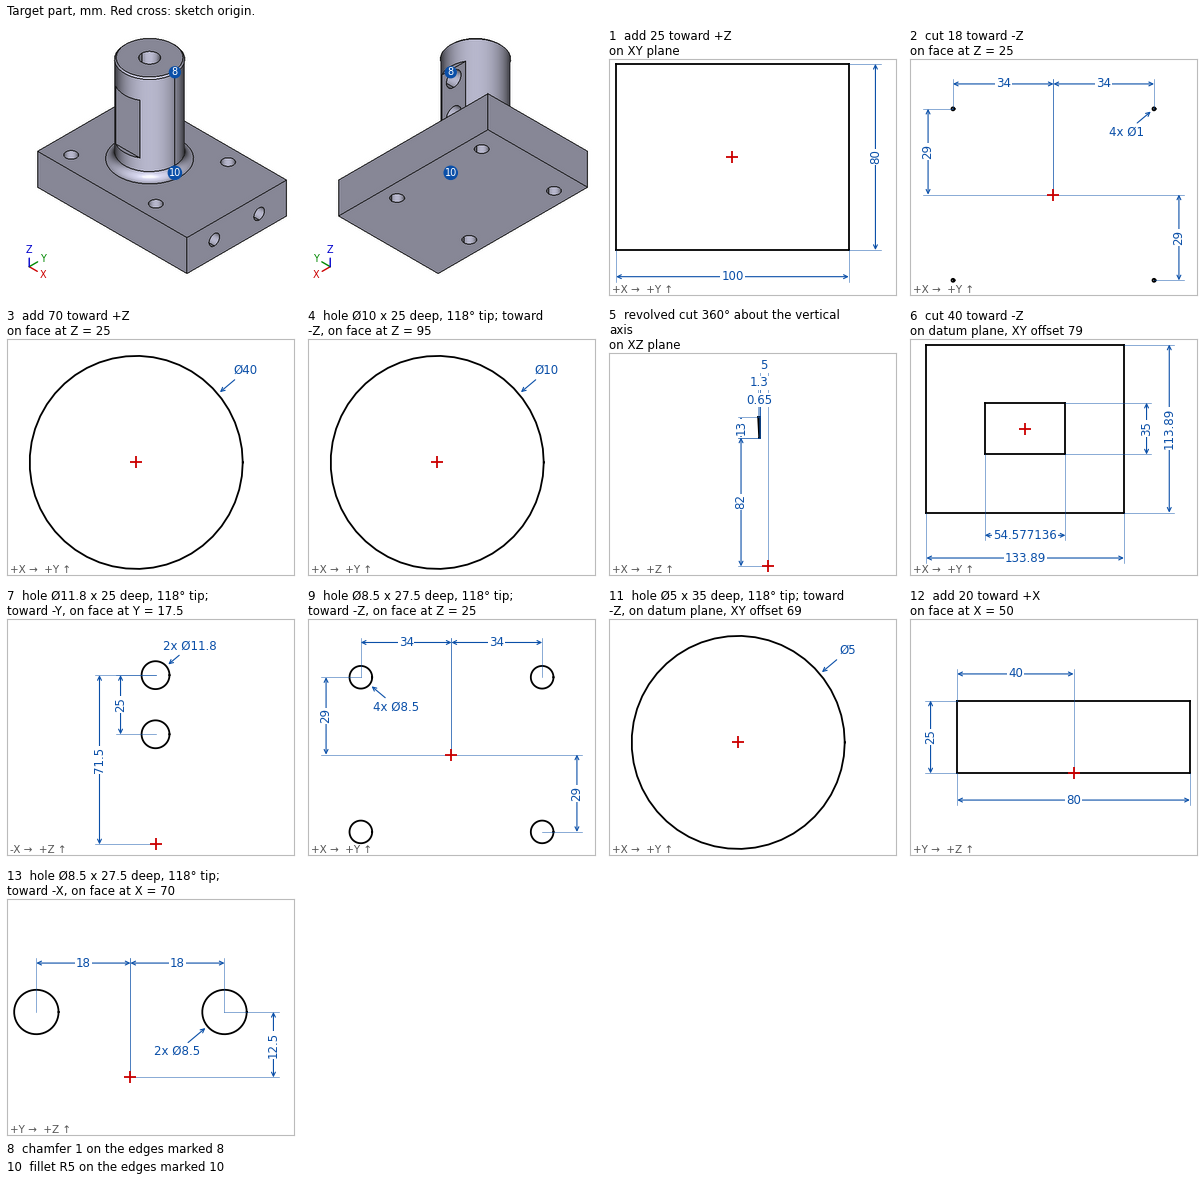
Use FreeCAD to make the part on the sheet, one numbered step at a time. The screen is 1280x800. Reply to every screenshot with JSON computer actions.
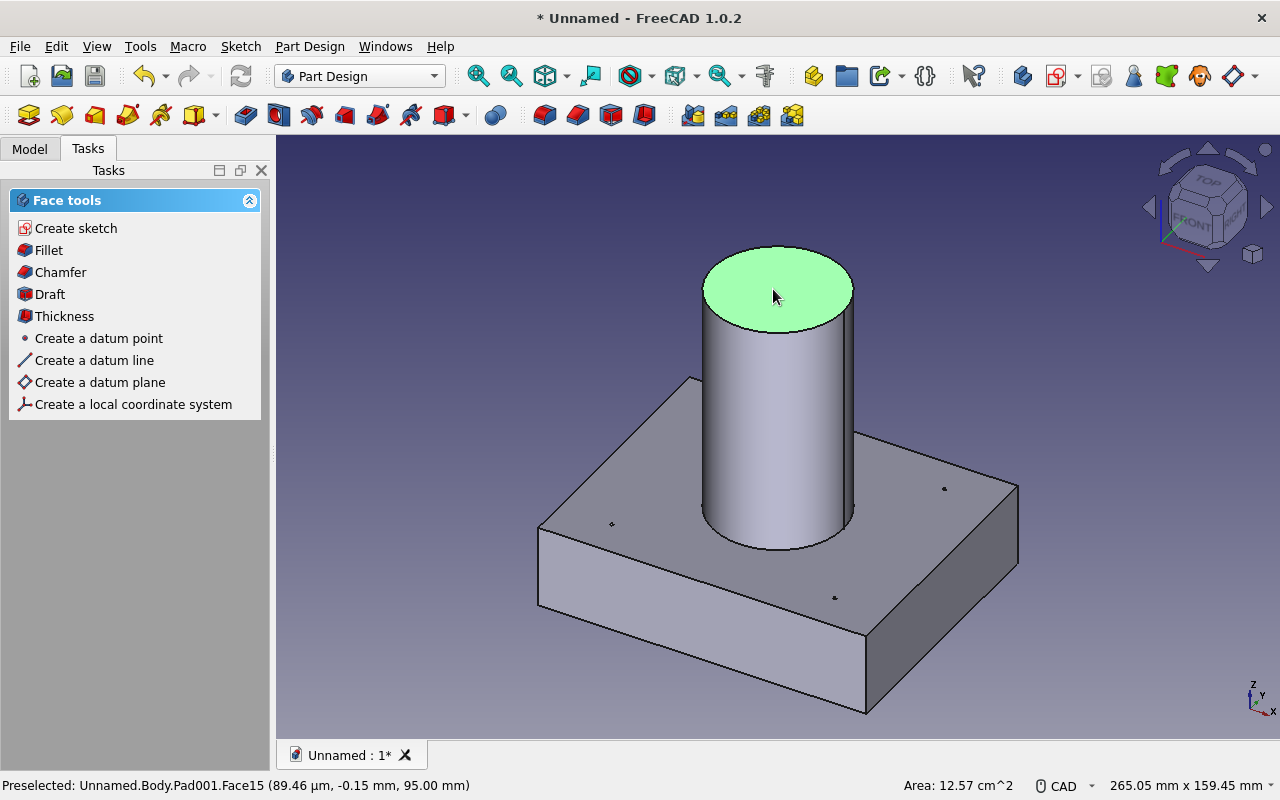
{"action": "left_click", "coordinate": [1056, 76]}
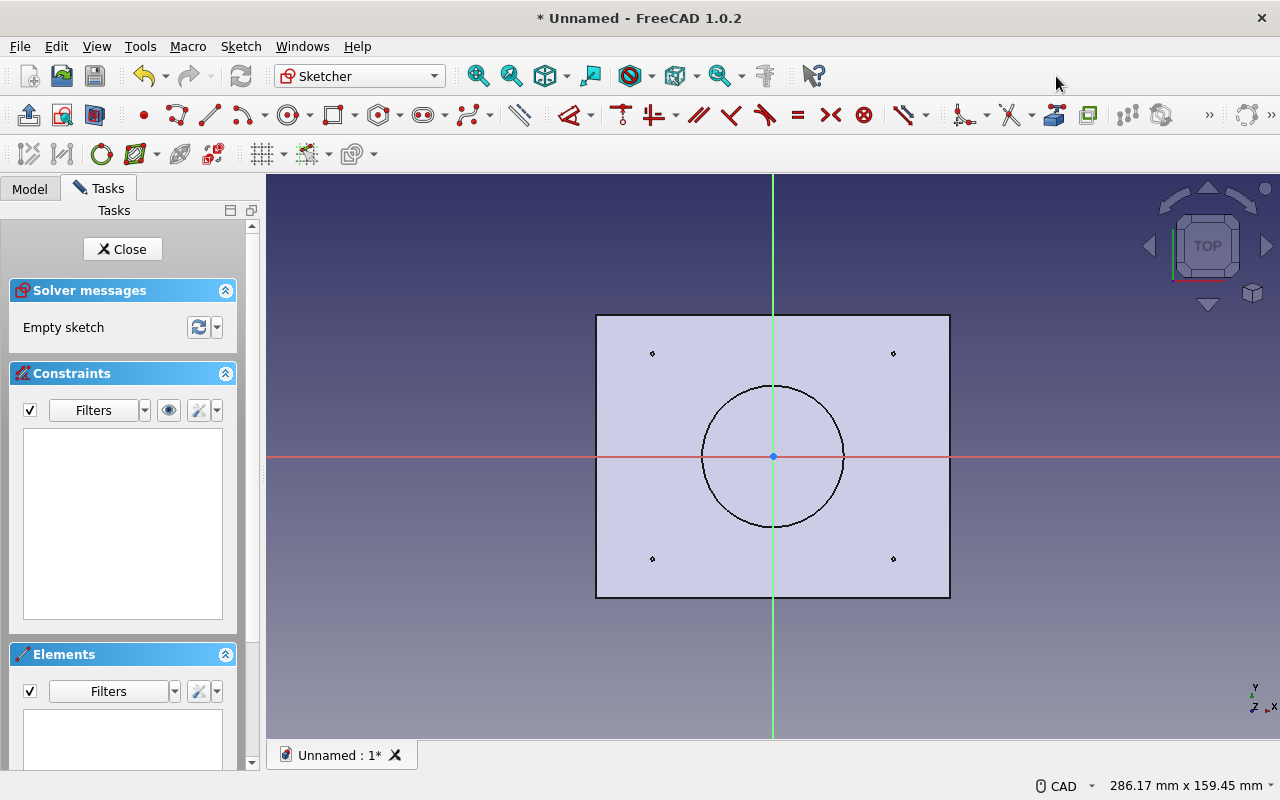
{"action": "scroll", "coordinate": [780, 456], "scroll_direction": "up", "scroll_amount": 12}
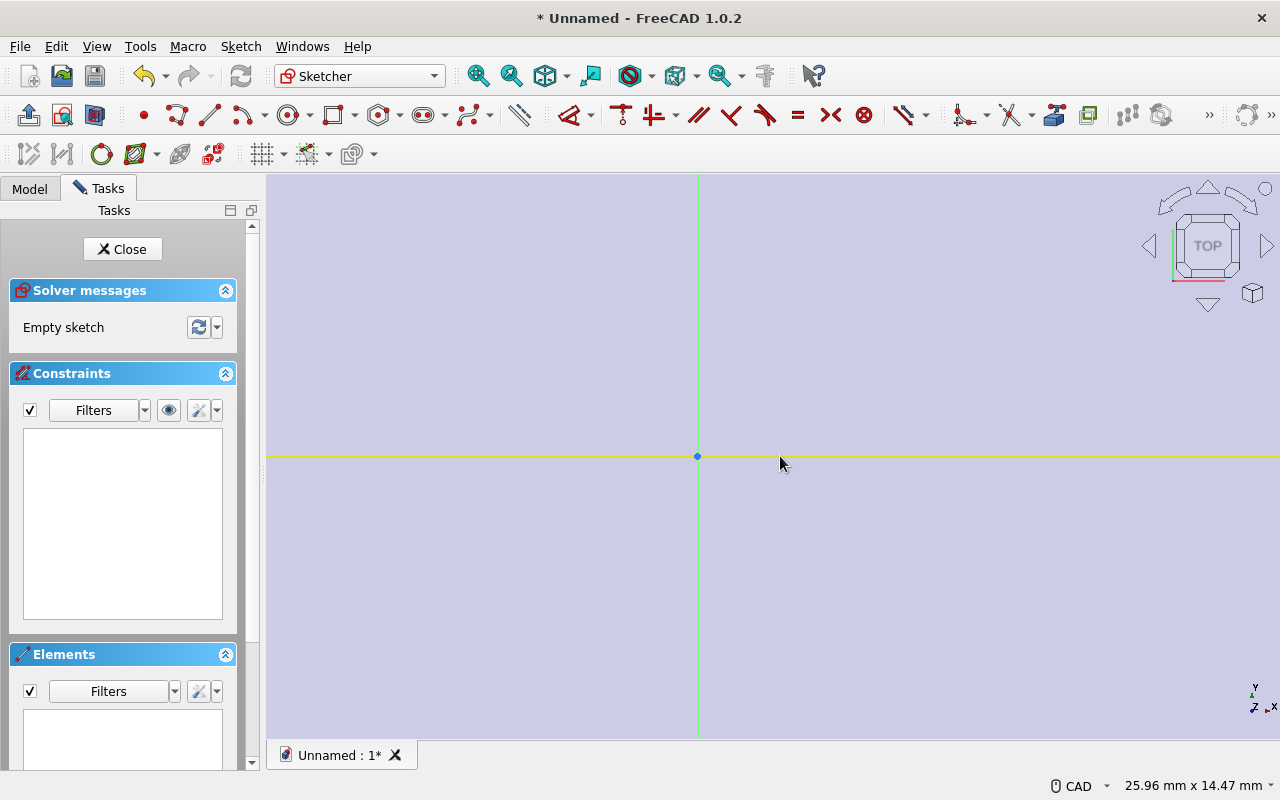
{"action": "key", "text": "g c"}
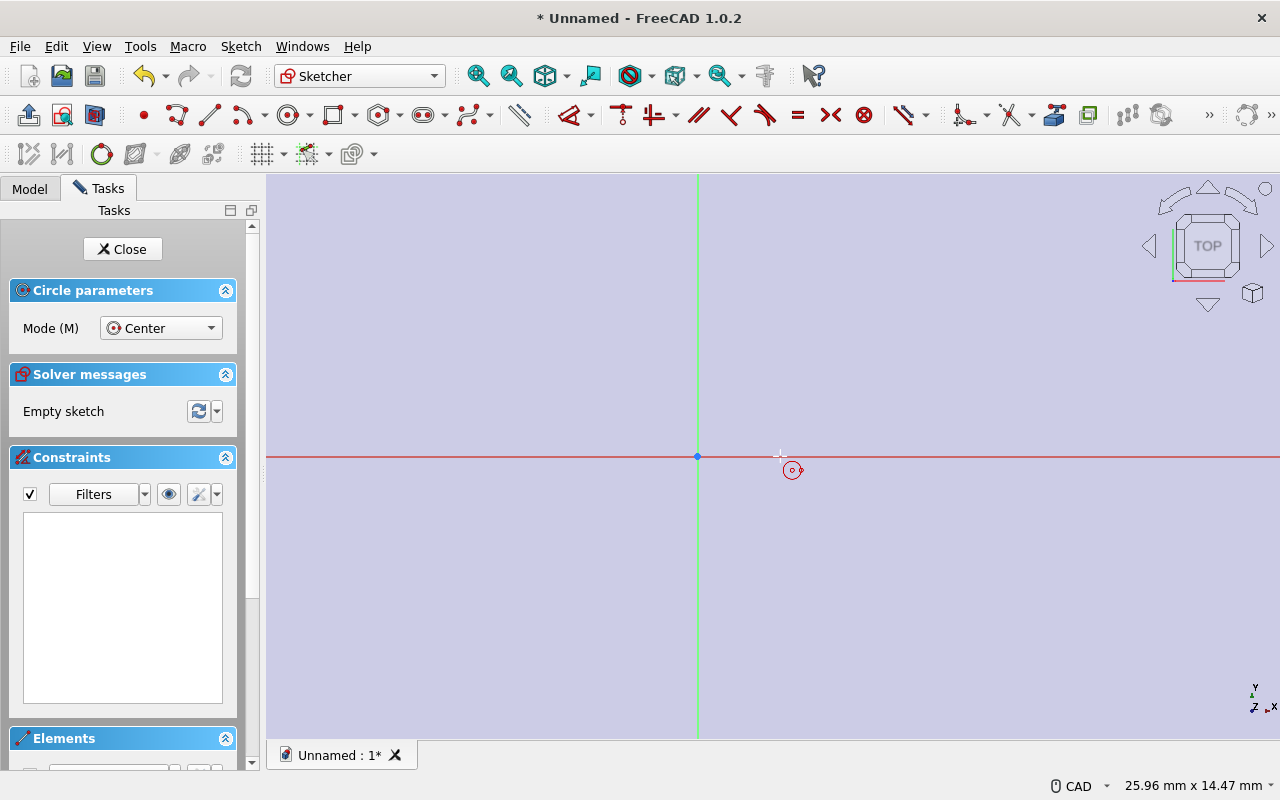
{"action": "left_click", "coordinate": [698, 456]}
{"action": "mouse_move", "coordinate": [836, 318]}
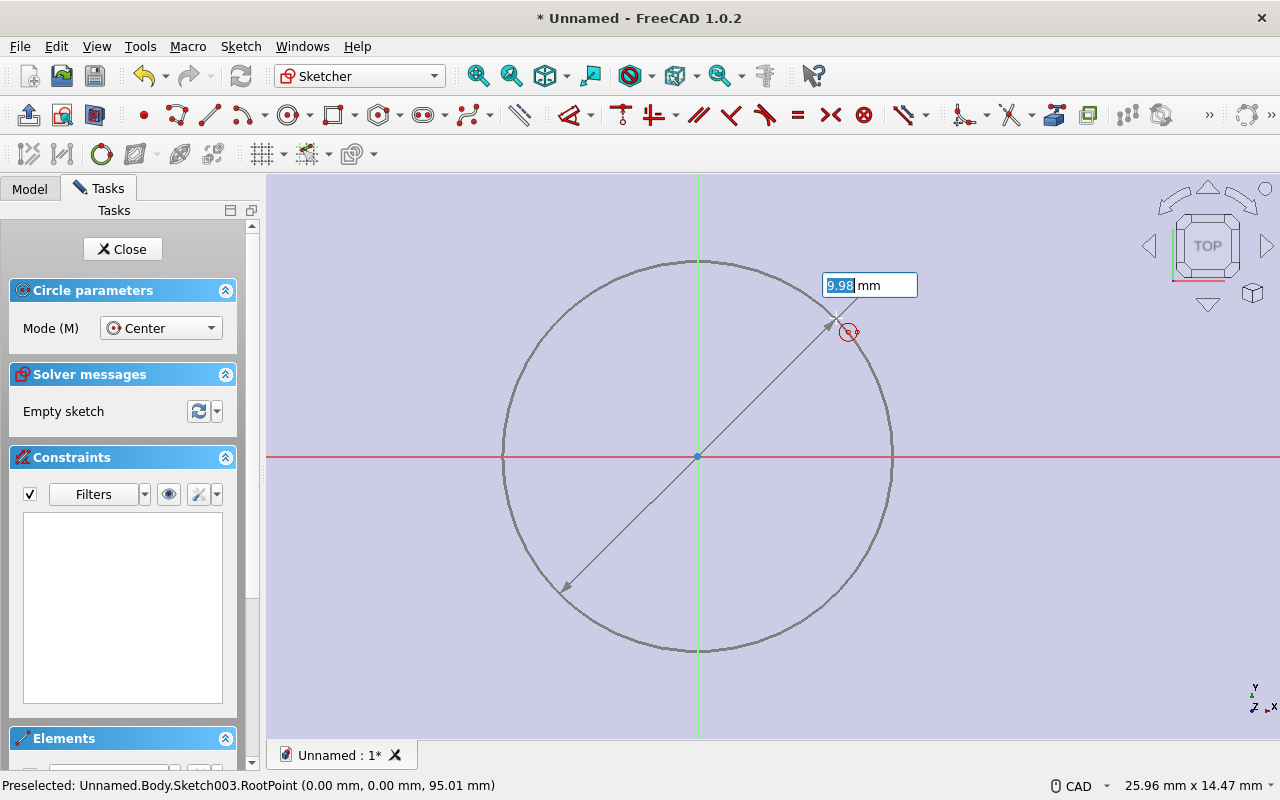
{"action": "type", "text": "10"}
{"action": "key", "text": "Return"}
{"action": "key", "text": "Escape"}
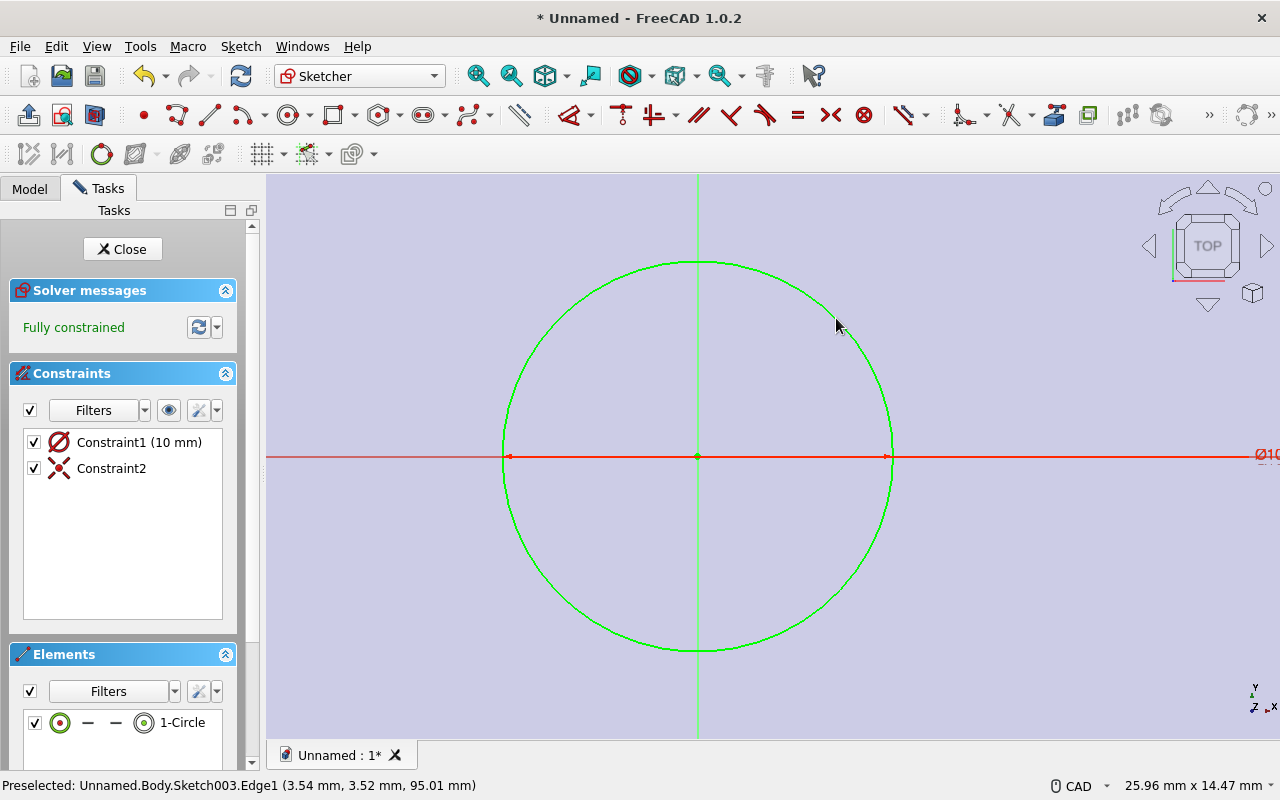
{"action": "left_click", "coordinate": [123, 249]}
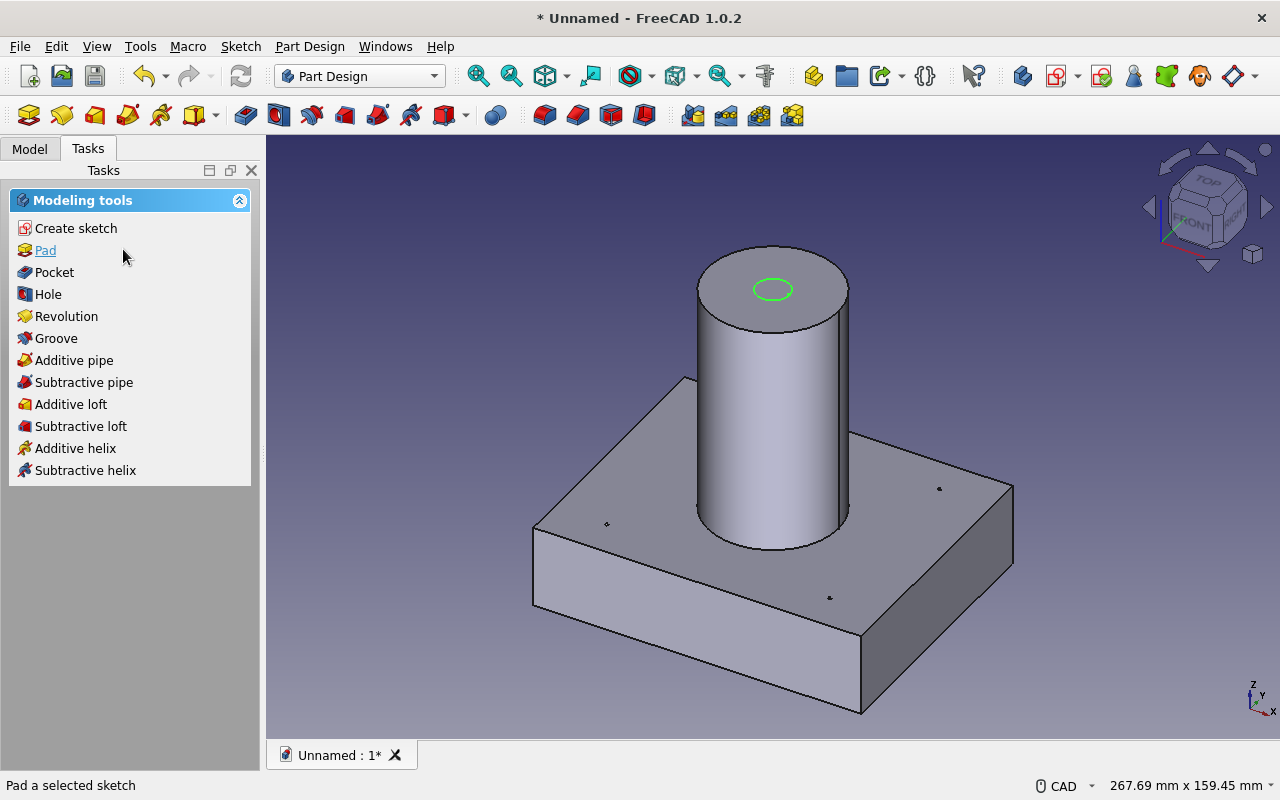
{"action": "left_click", "coordinate": [279, 116]}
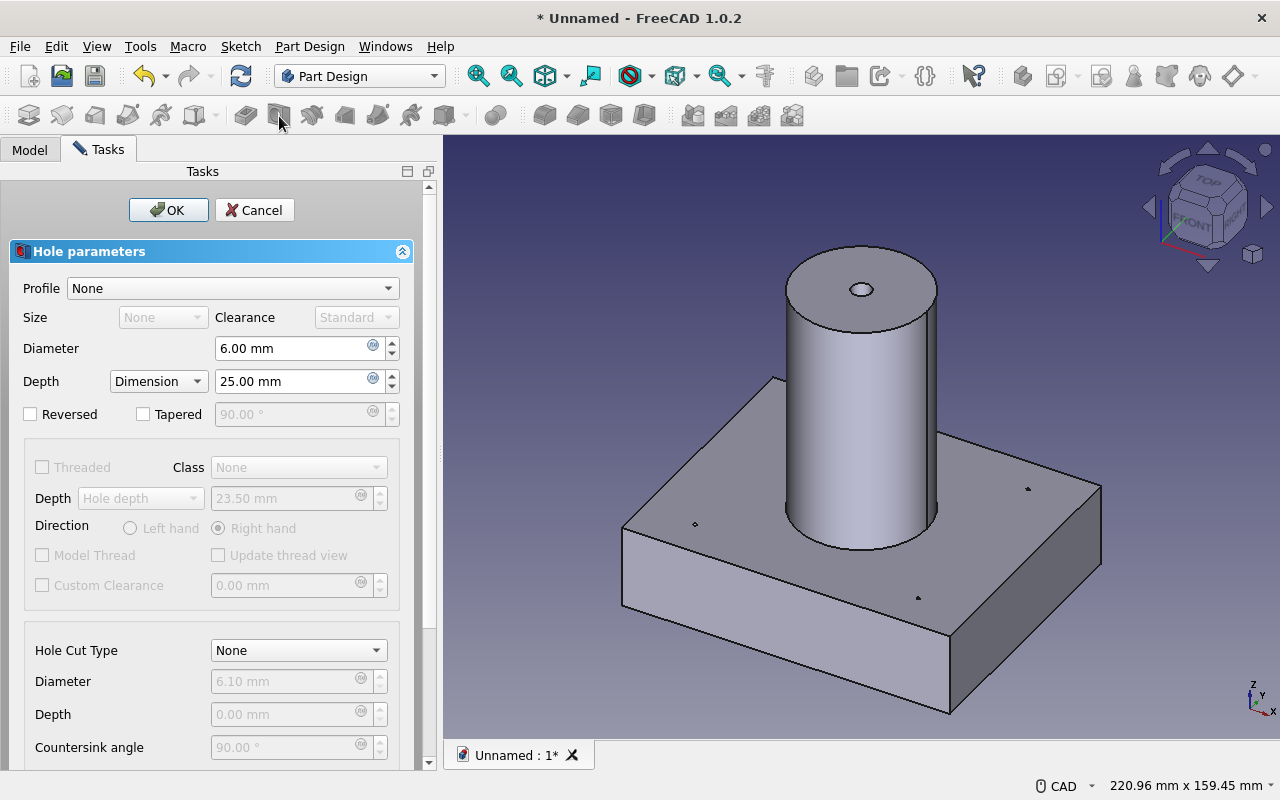
{"action": "triple_click", "coordinate": [300, 348]}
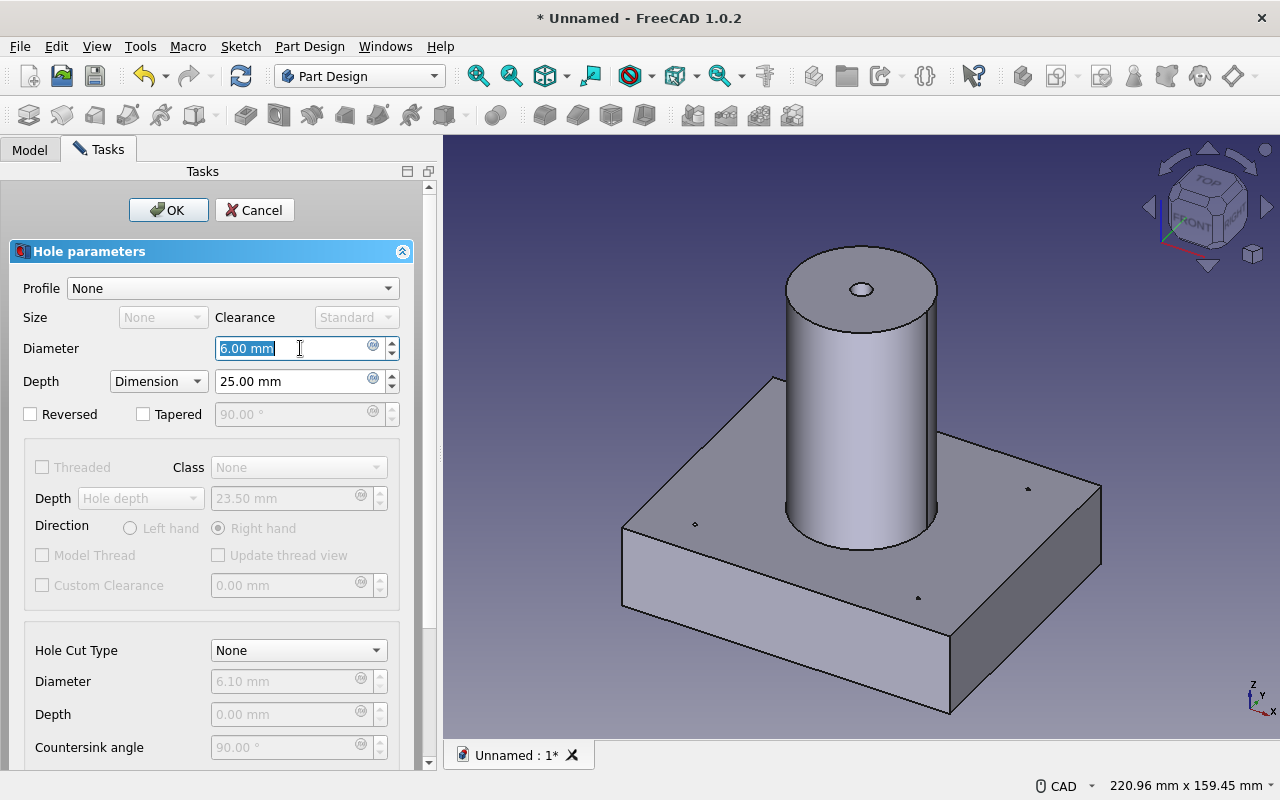
{"action": "type", "text": "10"}
{"action": "key", "text": "Tab"}